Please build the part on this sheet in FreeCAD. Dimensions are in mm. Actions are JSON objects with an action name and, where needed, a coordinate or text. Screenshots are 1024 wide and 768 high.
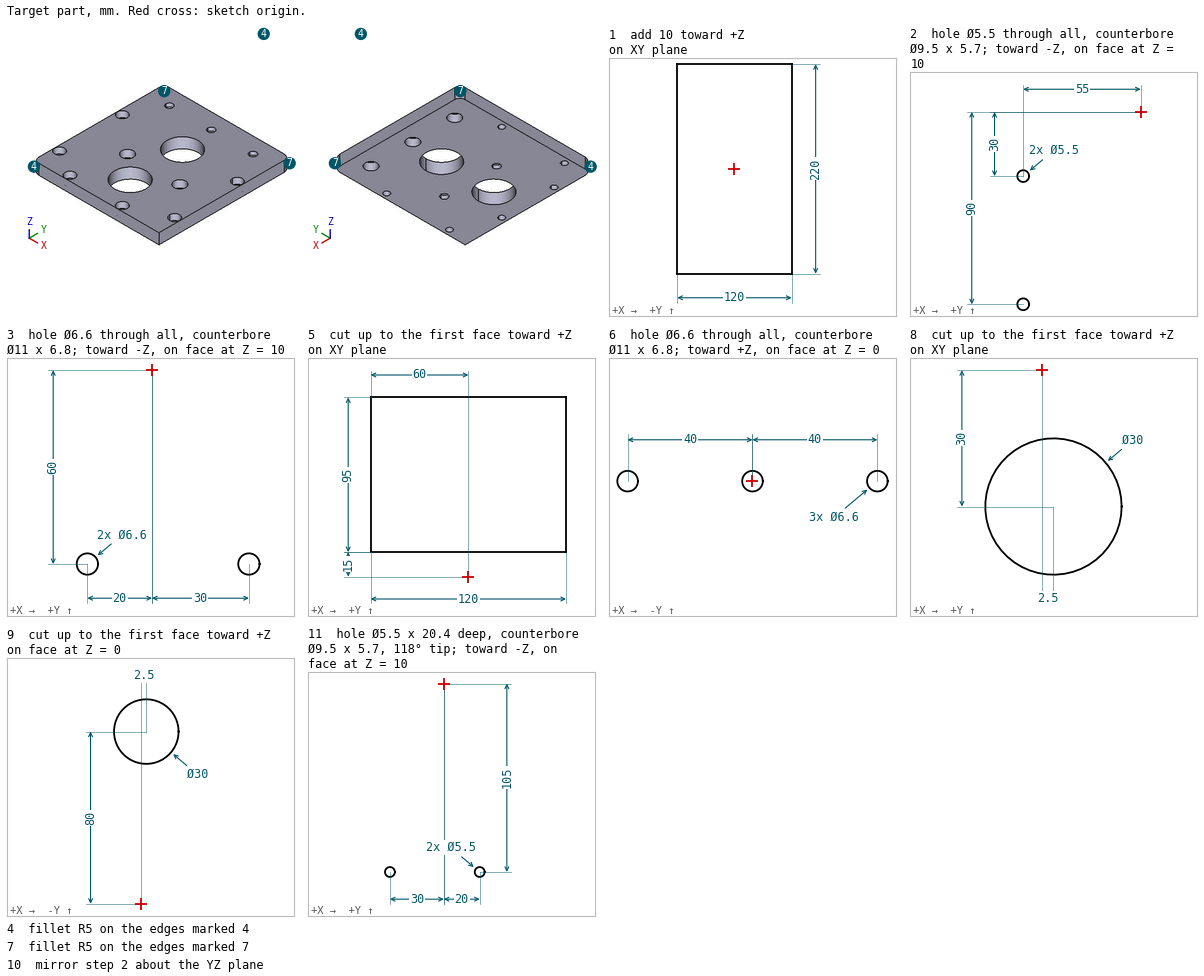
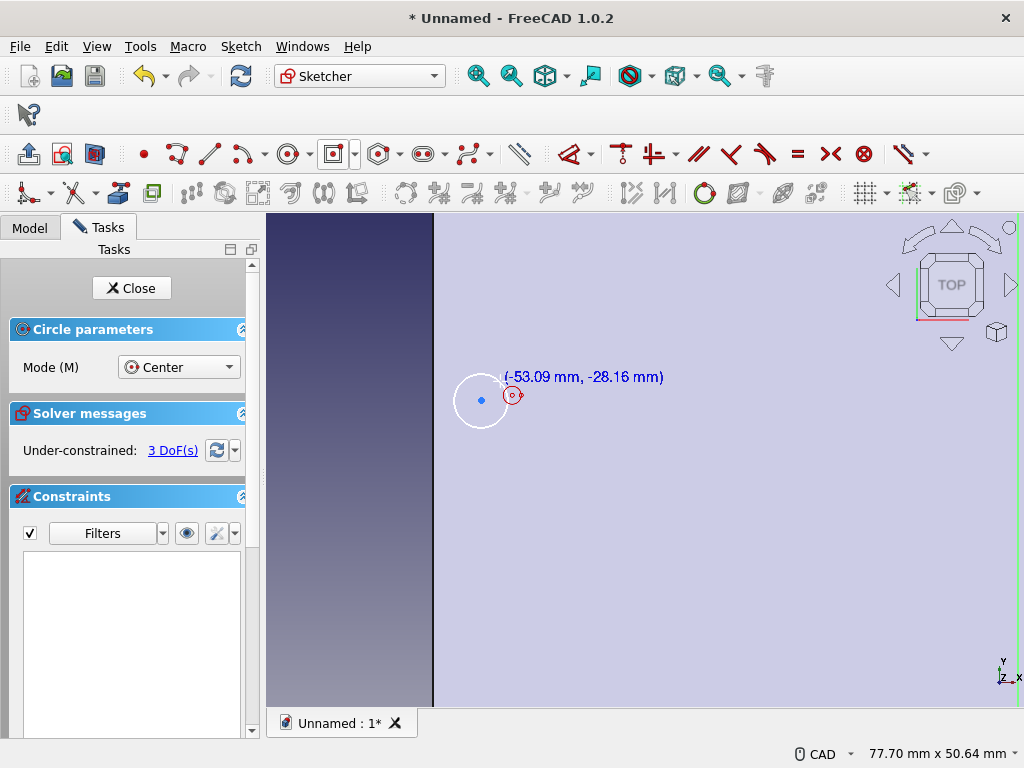
{"action": "scroll", "coordinate": [484, 402], "scroll_direction": "down", "scroll_amount": 5}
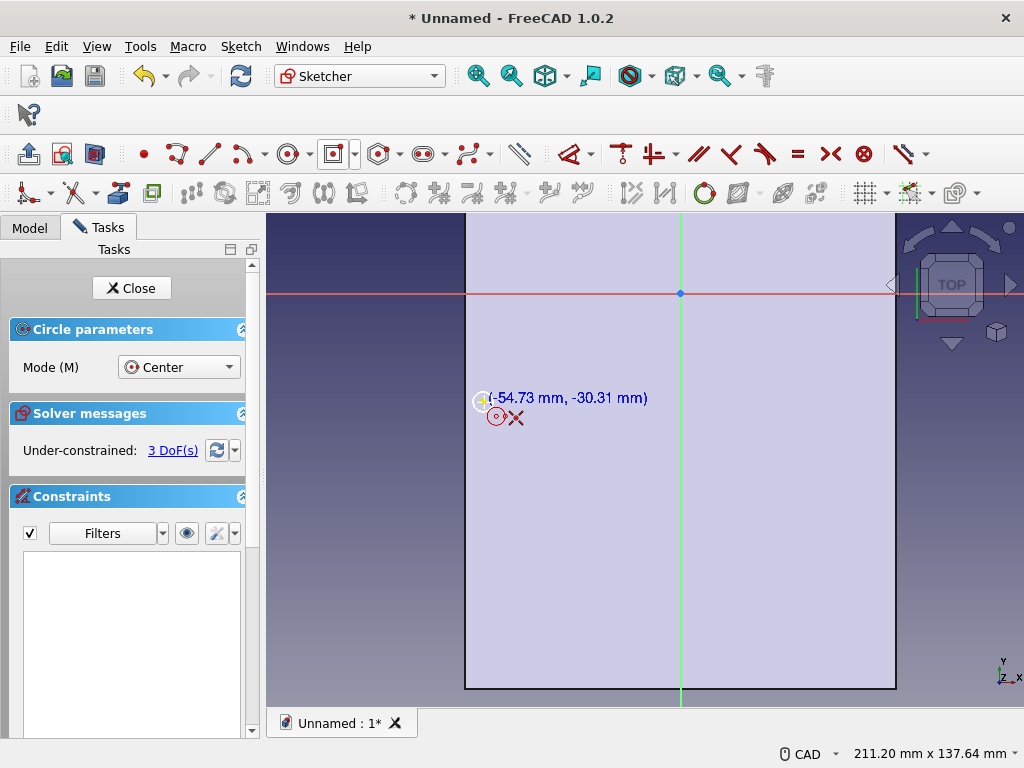
{"action": "scroll", "coordinate": [483, 617], "scroll_direction": "up", "scroll_amount": 5}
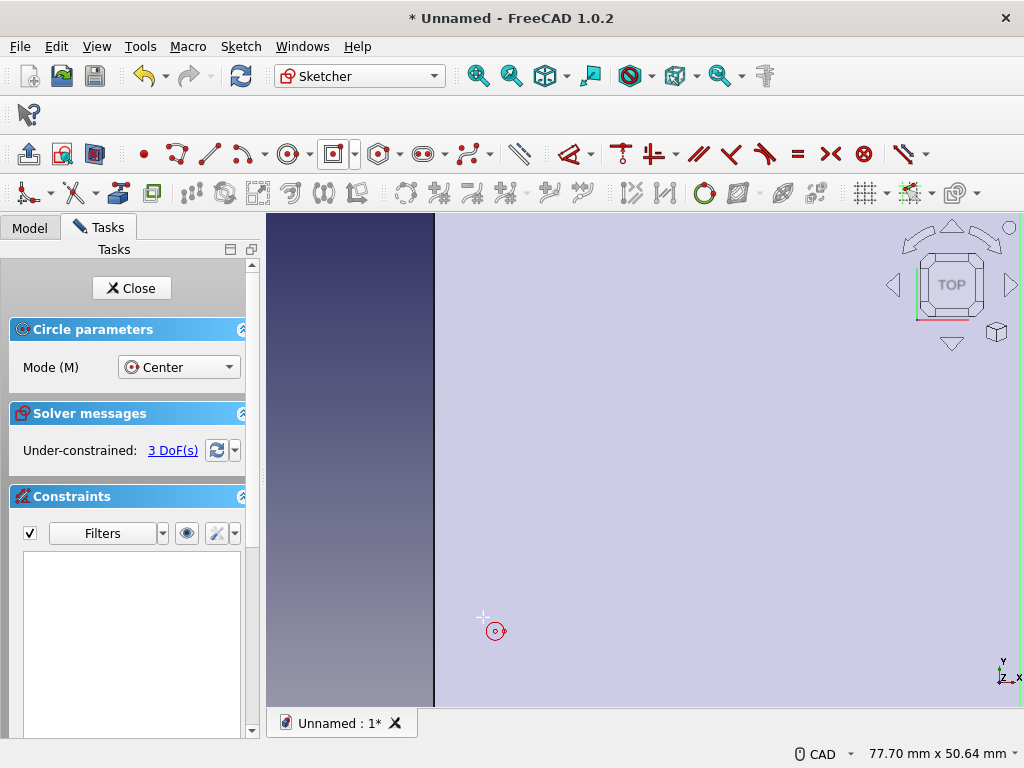
{"action": "left_click", "coordinate": [483, 615]}
{"action": "left_click", "coordinate": [502, 596]}
{"action": "key", "text": "Escape"}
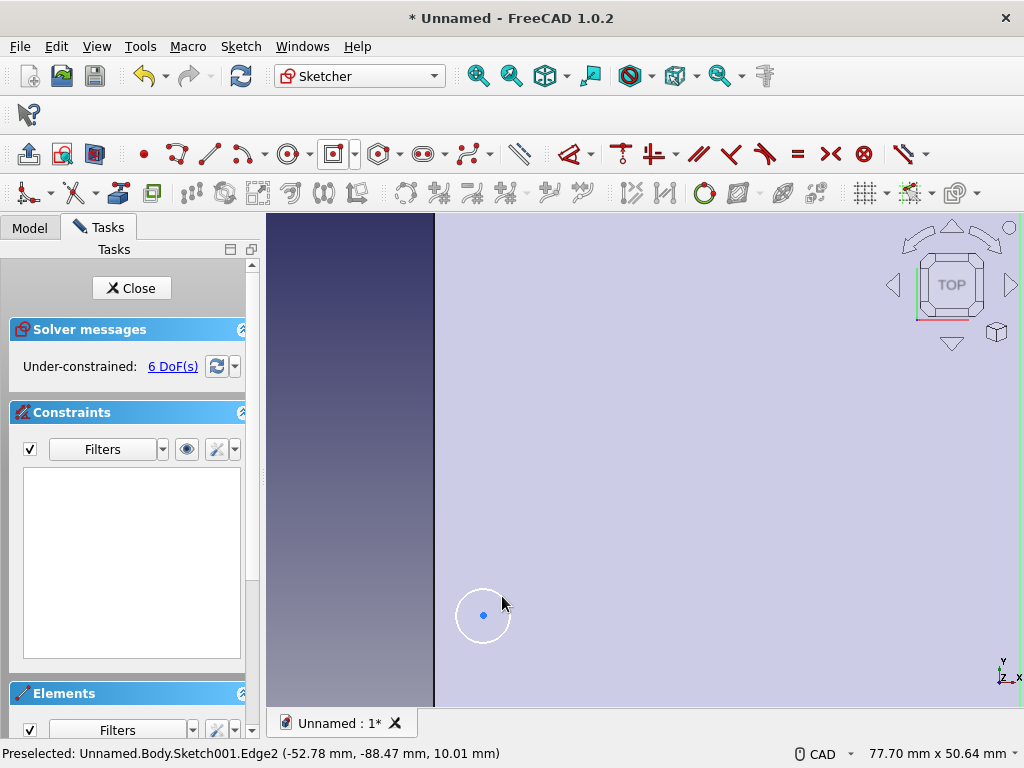
{"action": "scroll", "coordinate": [483, 617], "scroll_direction": "down", "scroll_amount": 5}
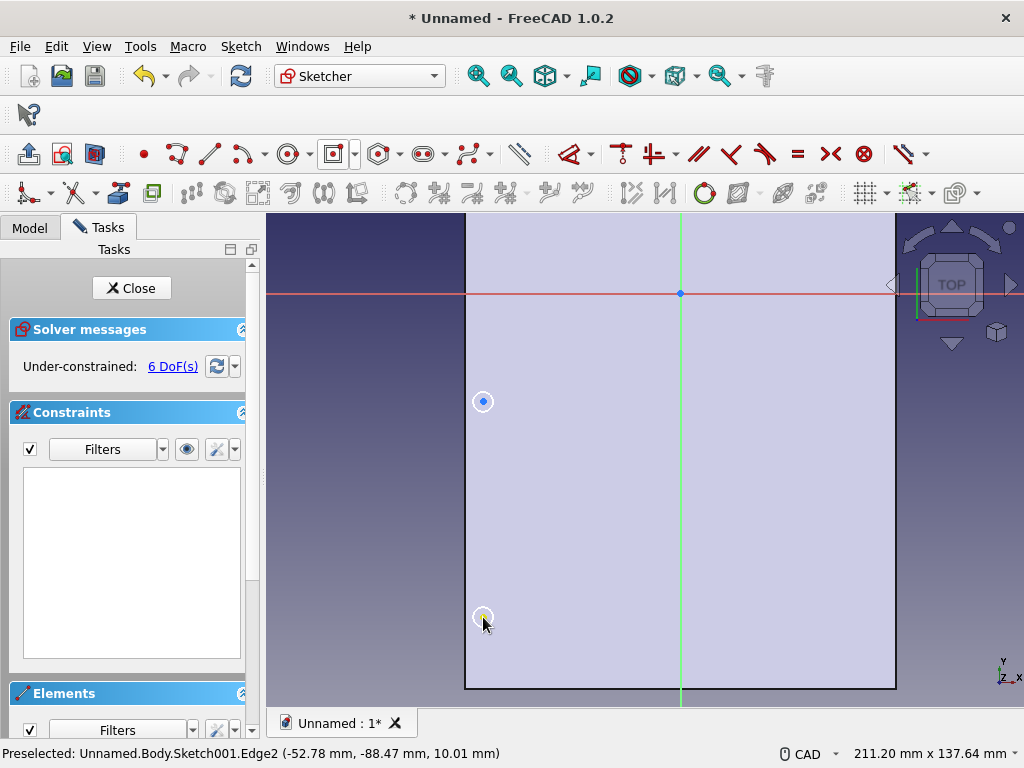
{"action": "scroll", "coordinate": [490, 395], "scroll_direction": "up", "scroll_amount": 2}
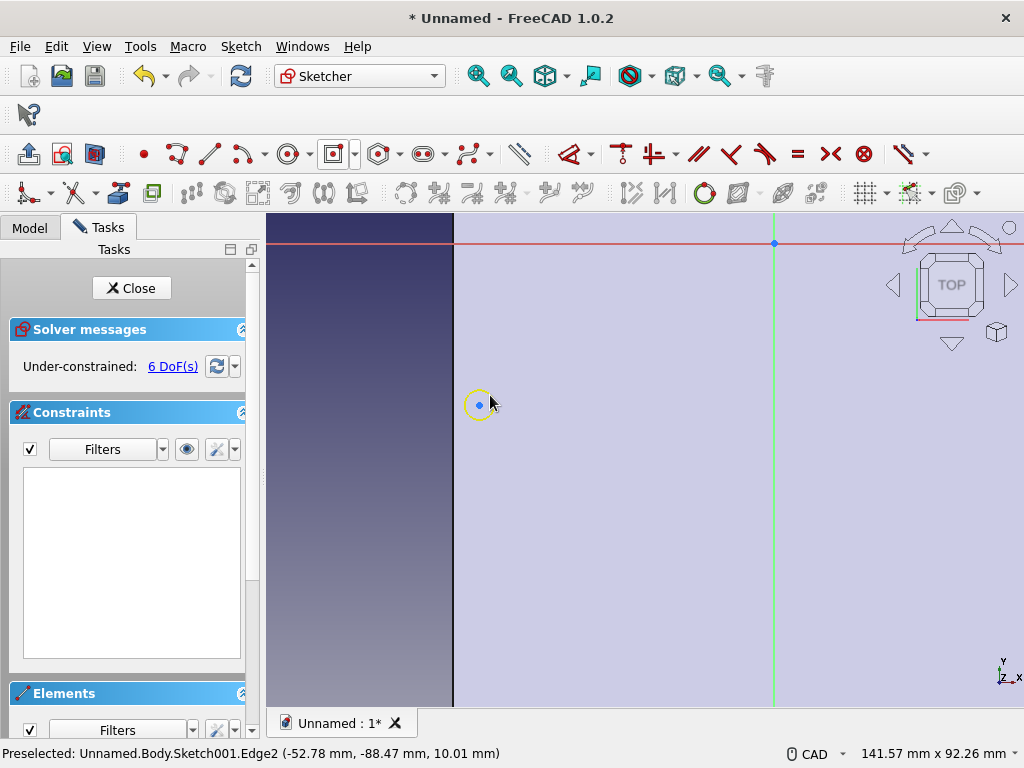
{"action": "left_click", "coordinate": [490, 395]}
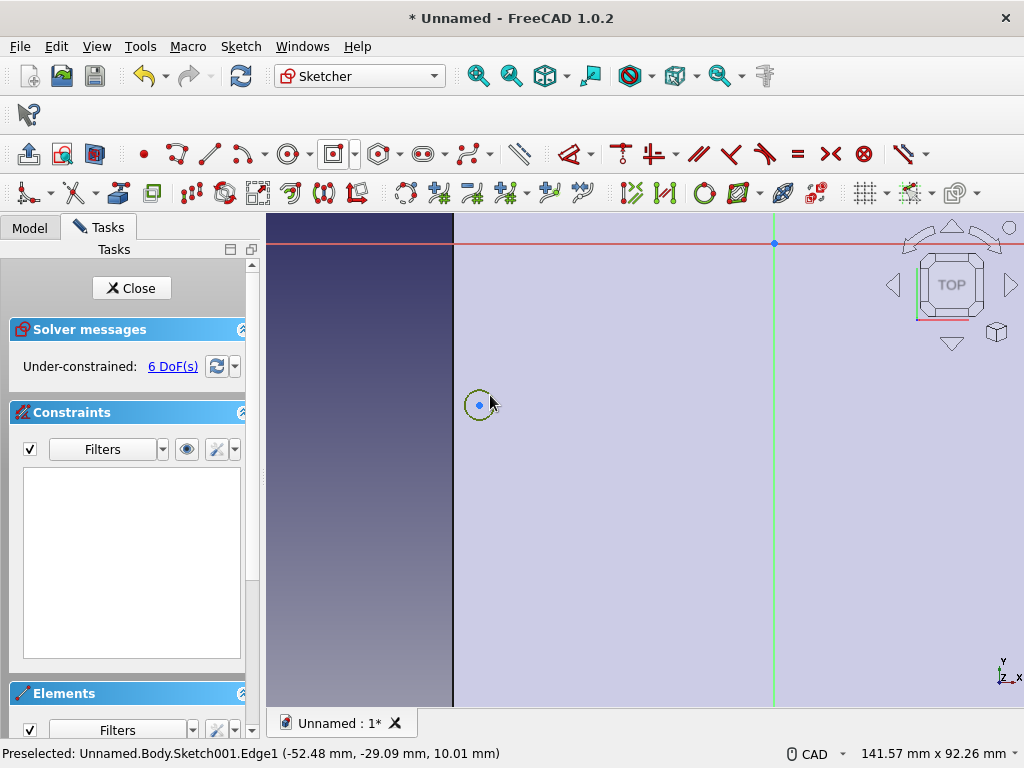
{"action": "scroll", "coordinate": [489, 395], "scroll_direction": "down", "scroll_amount": 2}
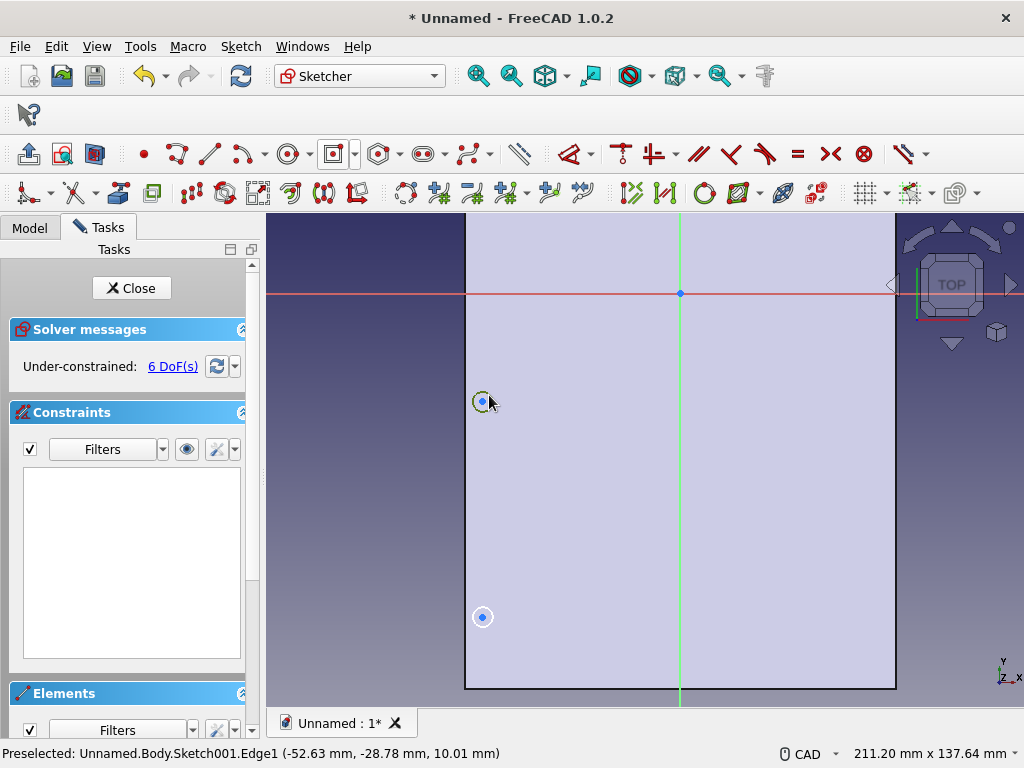
{"action": "scroll", "coordinate": [490, 610], "scroll_direction": "up", "scroll_amount": 2}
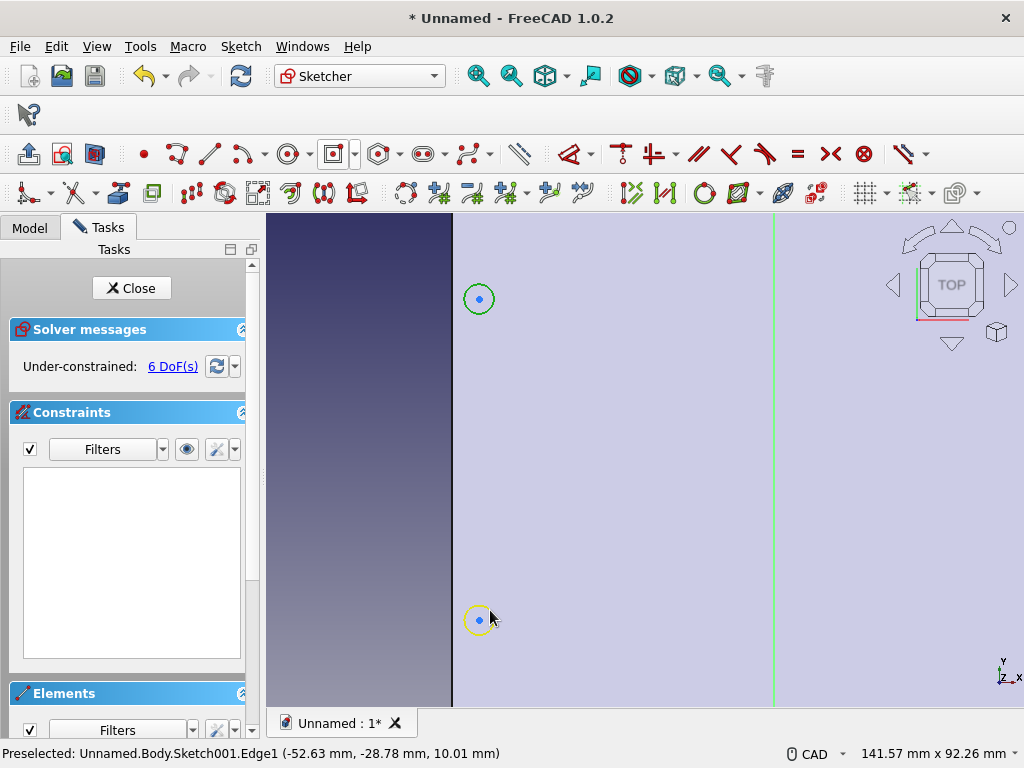
{"action": "left_click", "coordinate": [490, 610]}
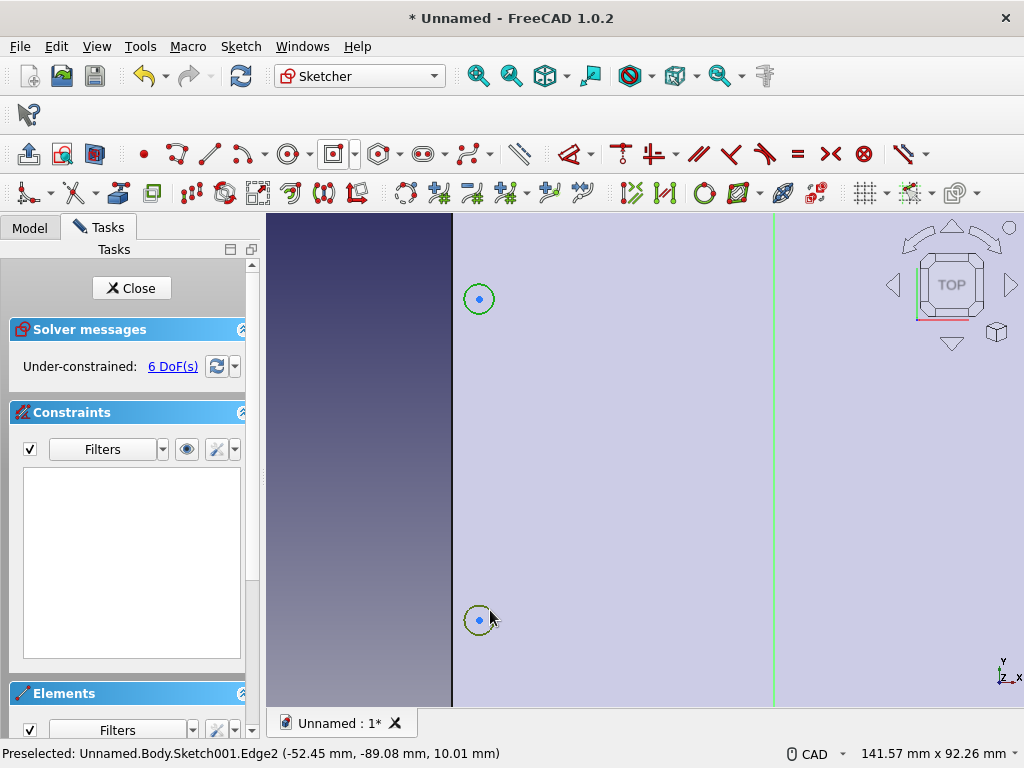
{"action": "left_click", "coordinate": [798, 154]}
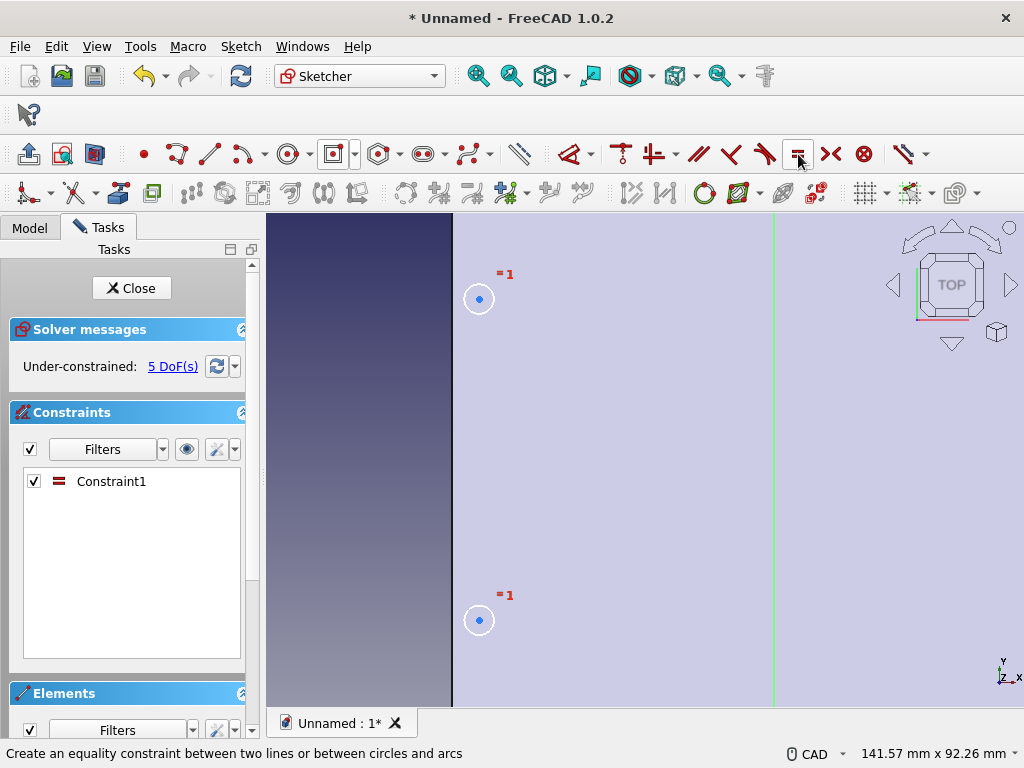
{"action": "left_click", "coordinate": [479, 299]}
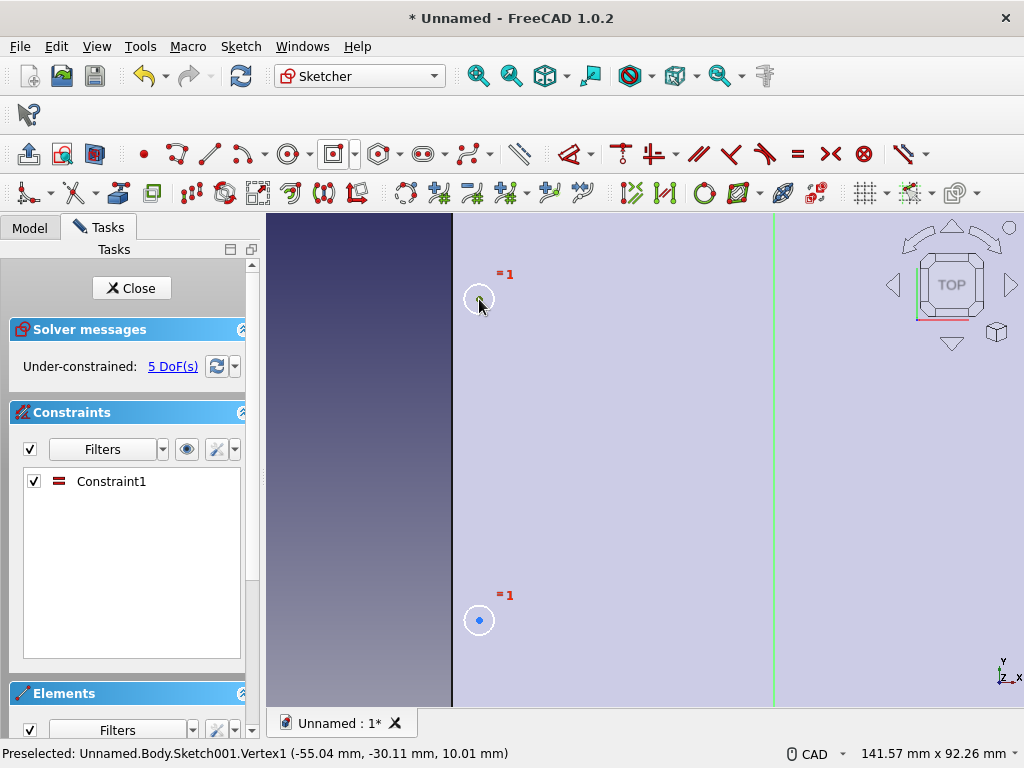
{"action": "left_click", "coordinate": [479, 620]}